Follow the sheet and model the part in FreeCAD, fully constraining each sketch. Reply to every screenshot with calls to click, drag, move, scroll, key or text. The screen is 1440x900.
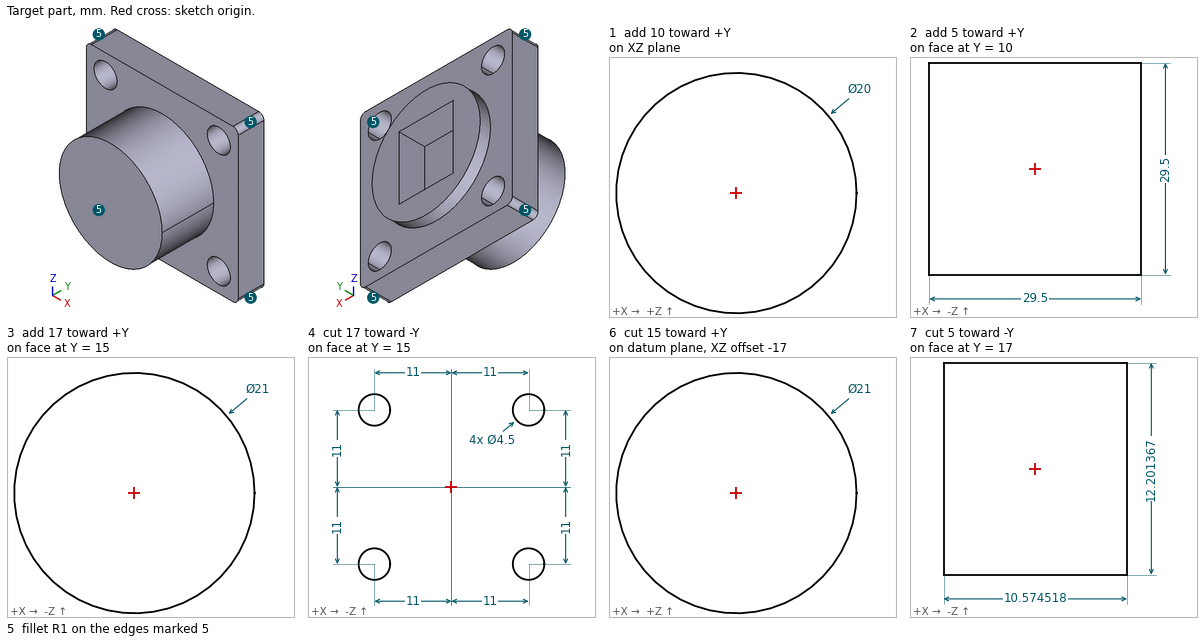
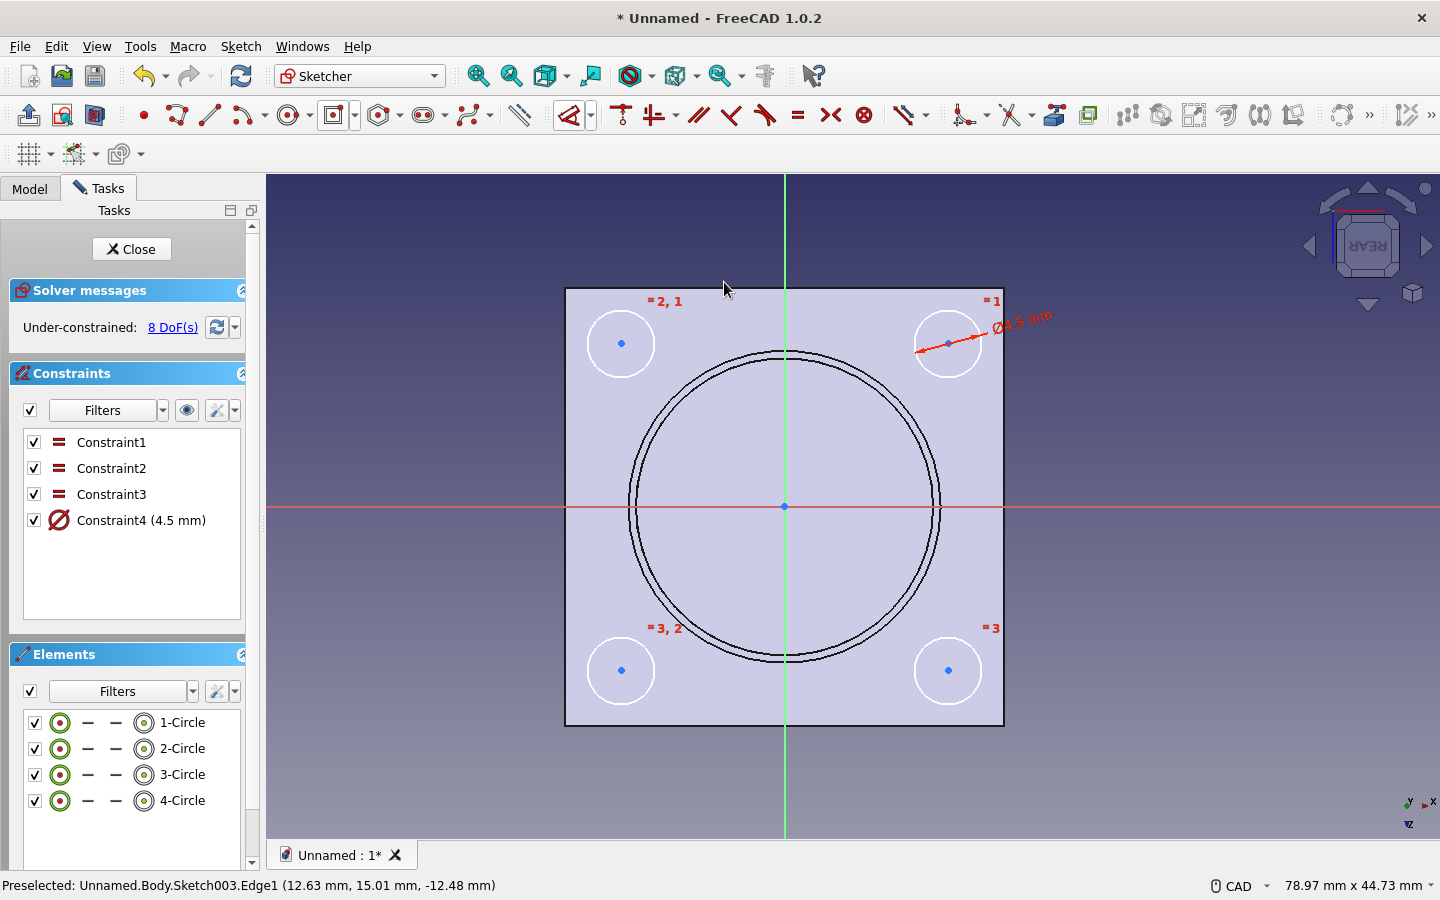
click(948, 344)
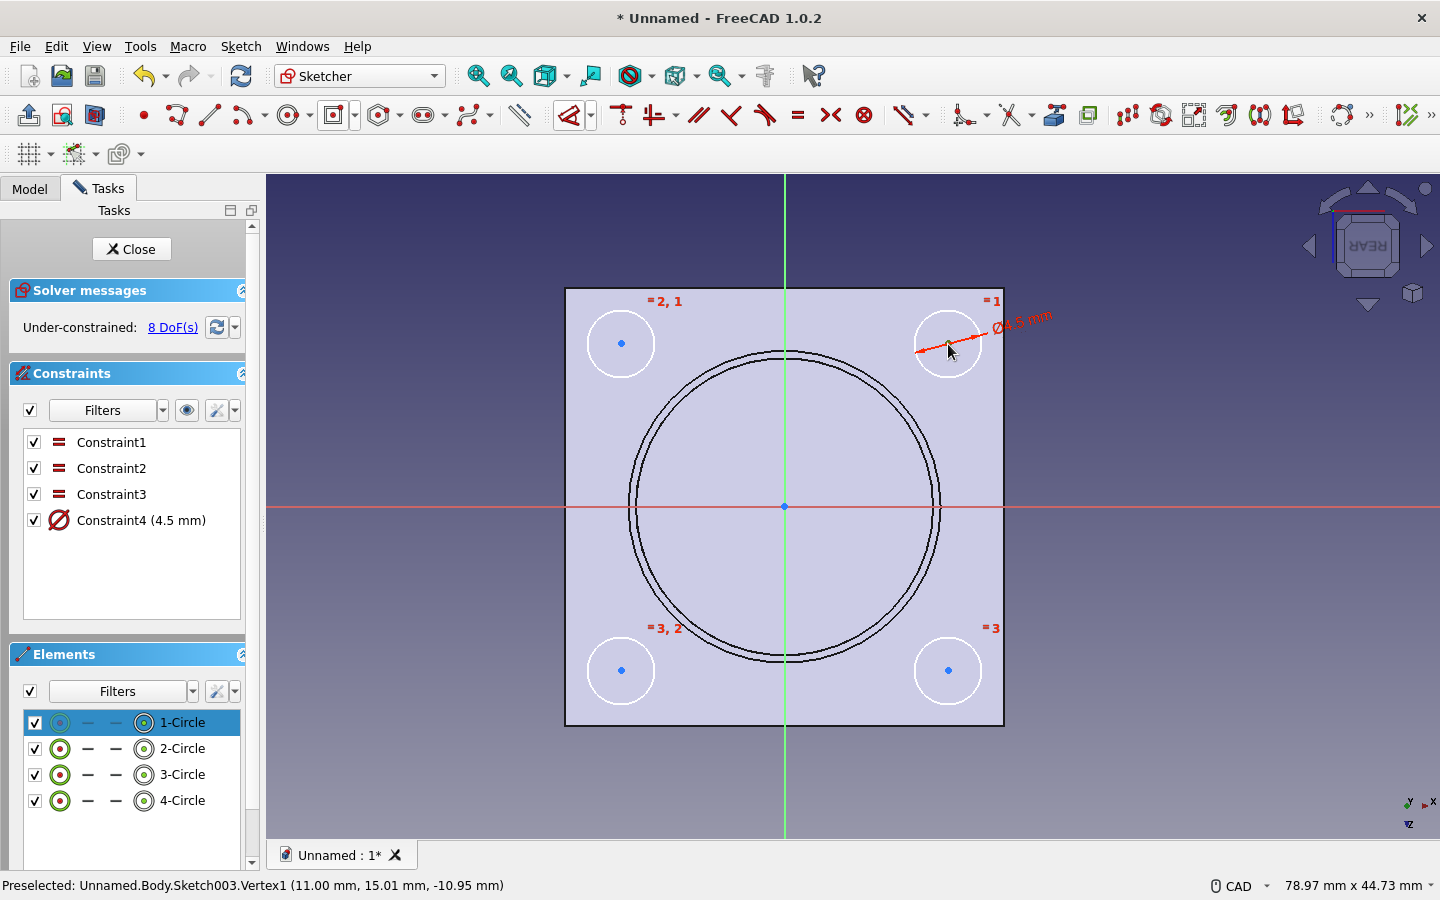
click(590, 116)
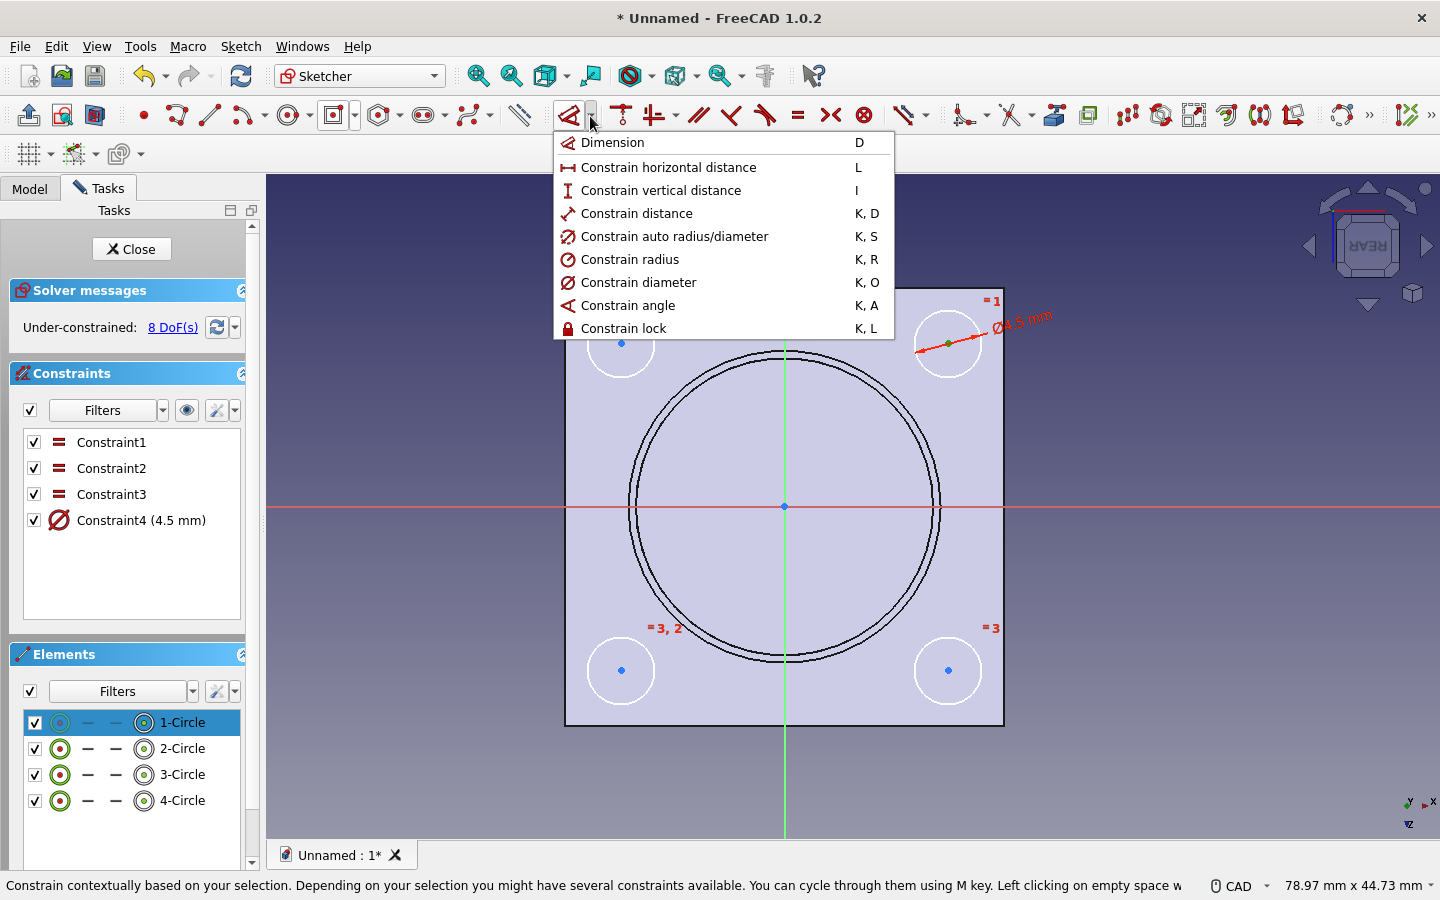
click(724, 168)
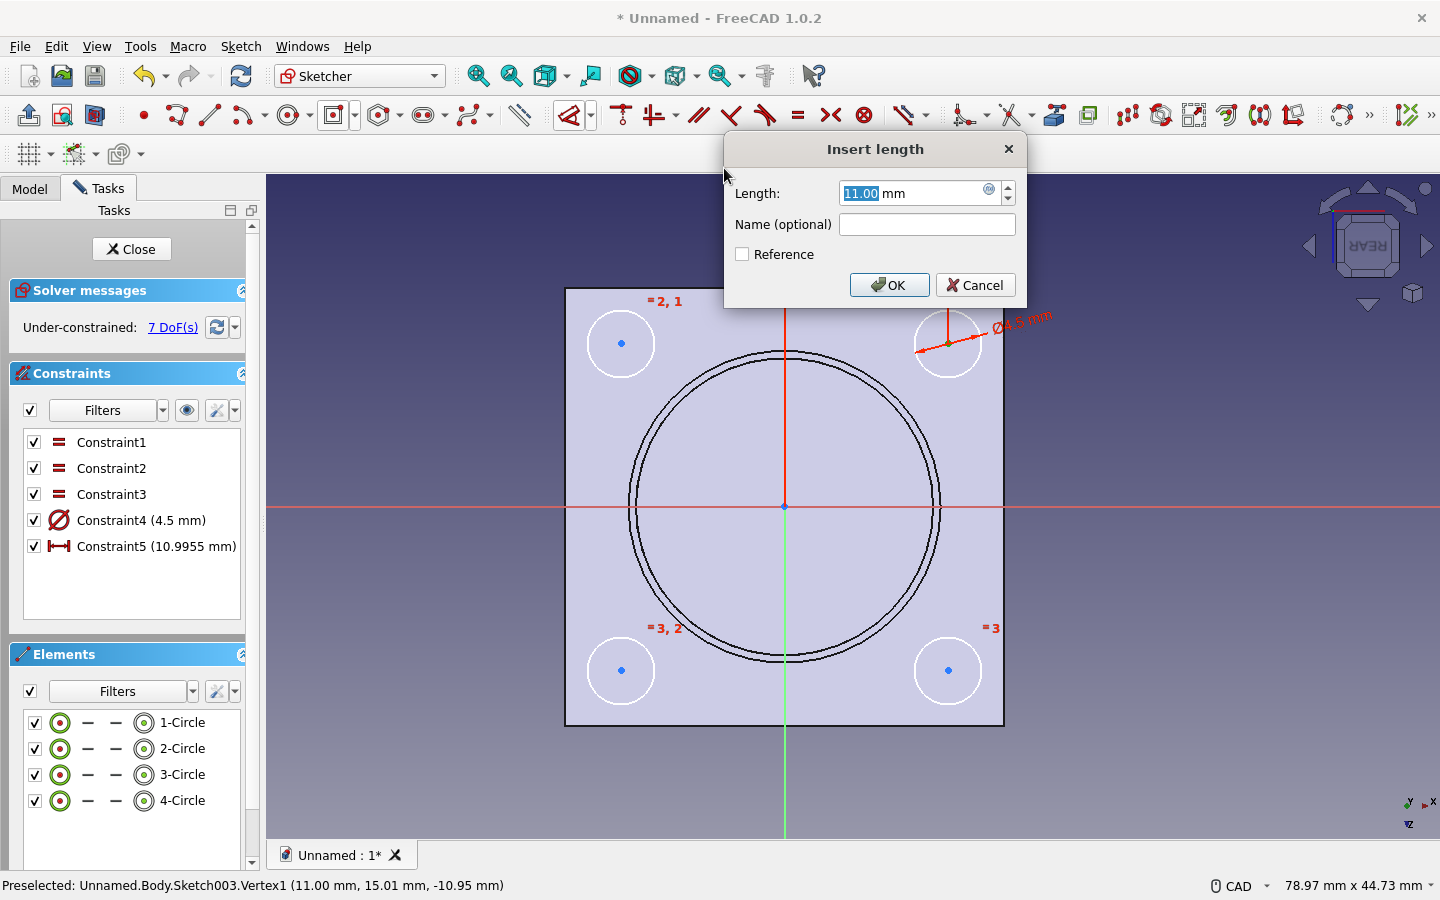
text(11)
key(Return)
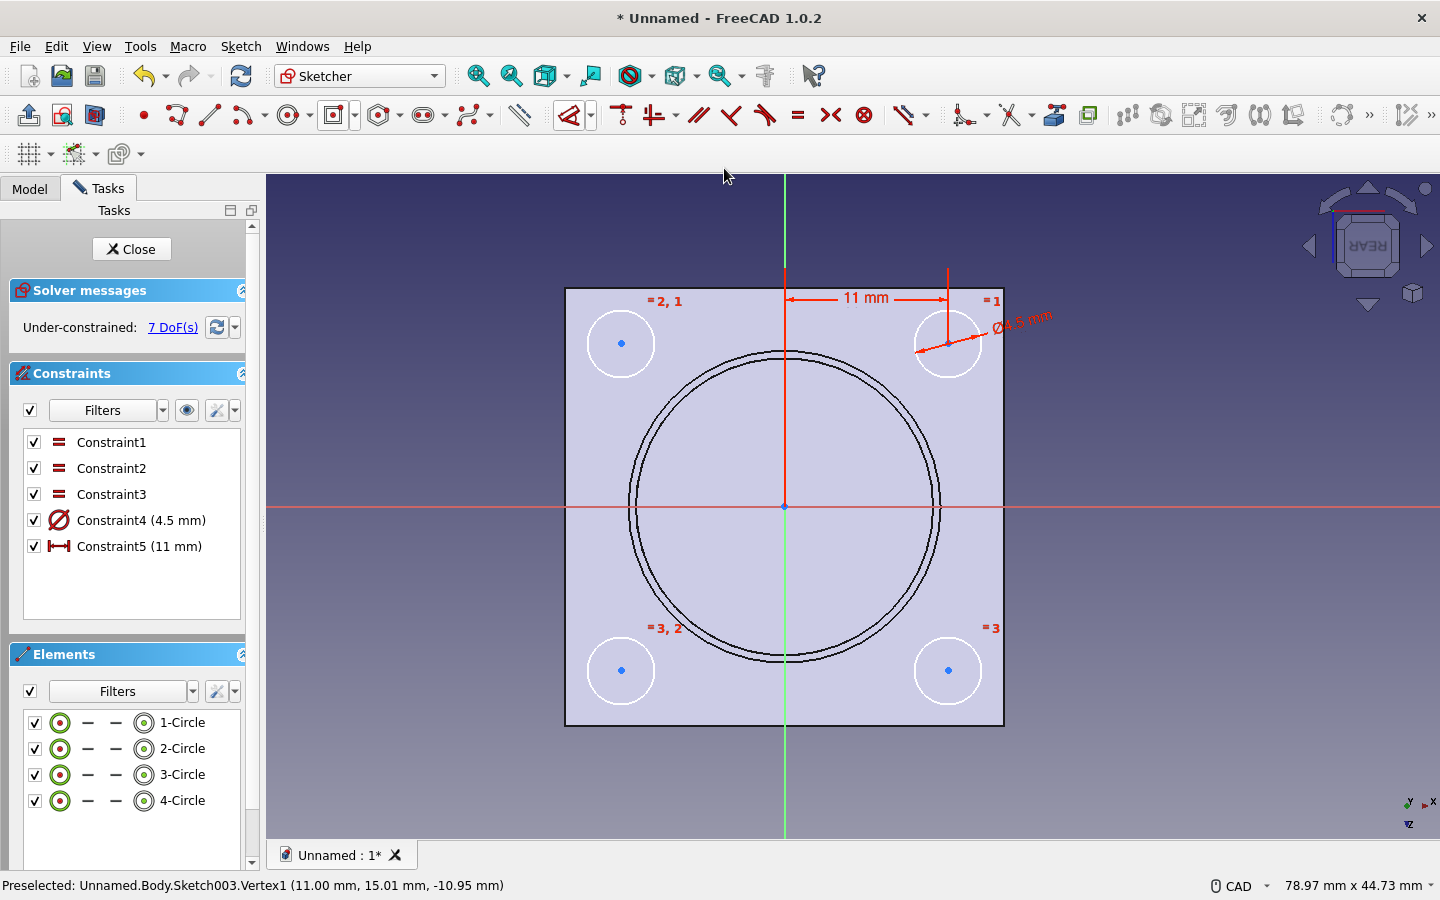
click(948, 344)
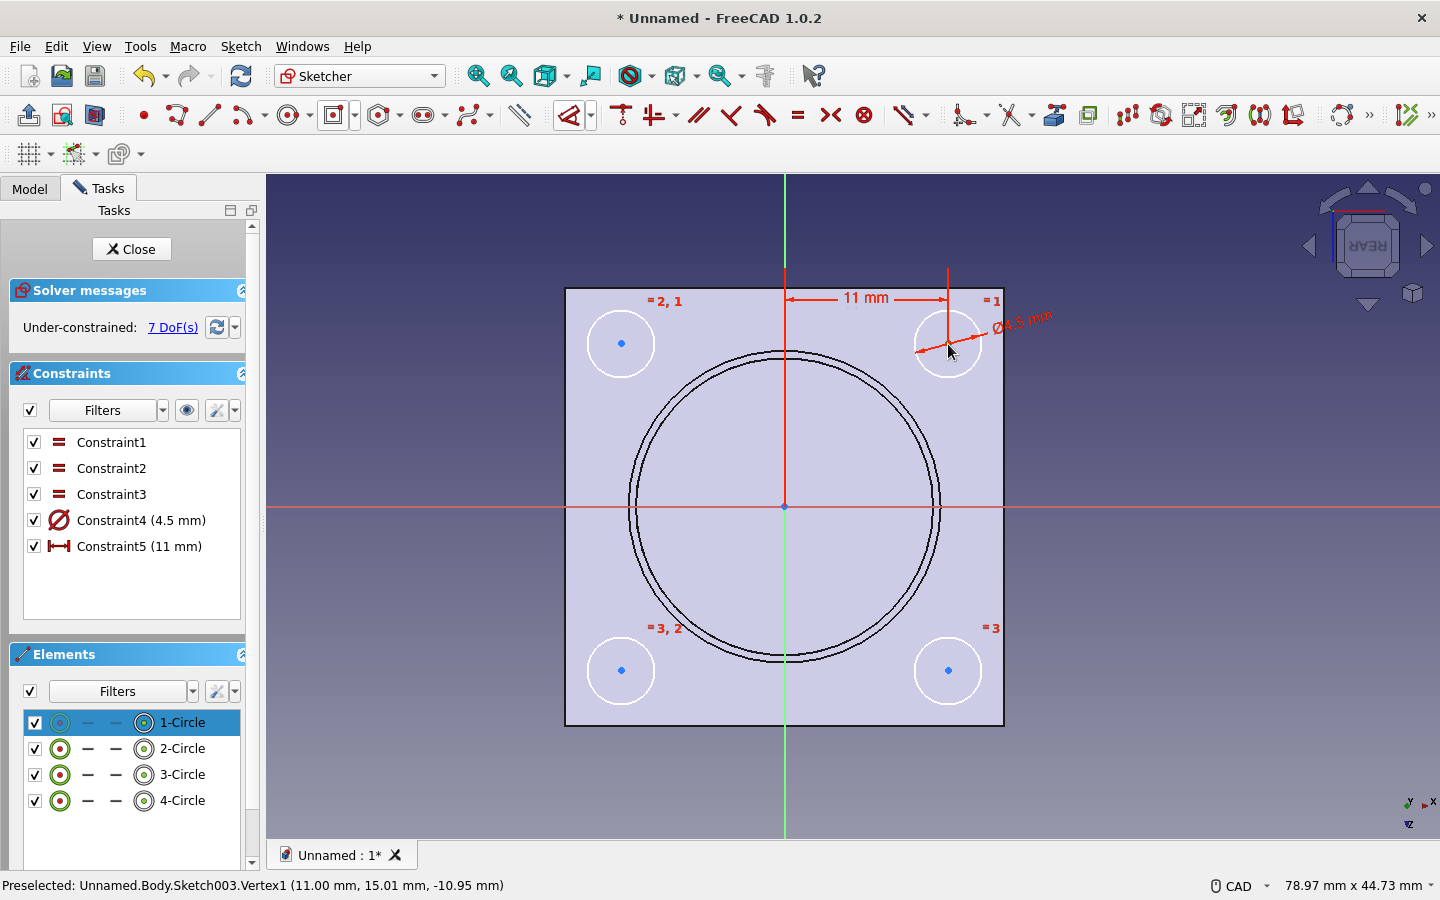
key(i)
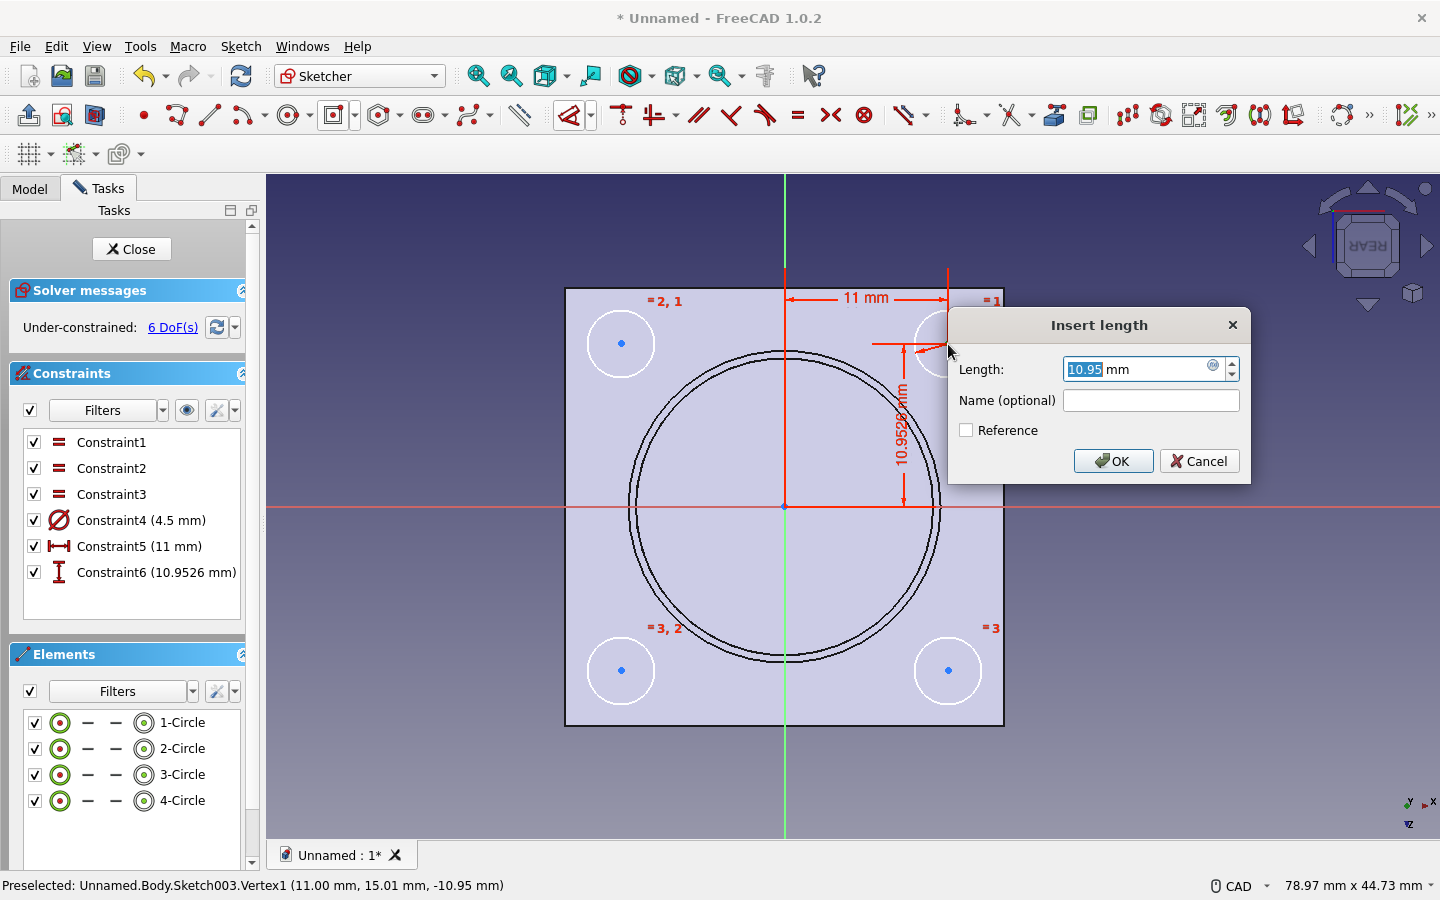
text(11)
key(Return)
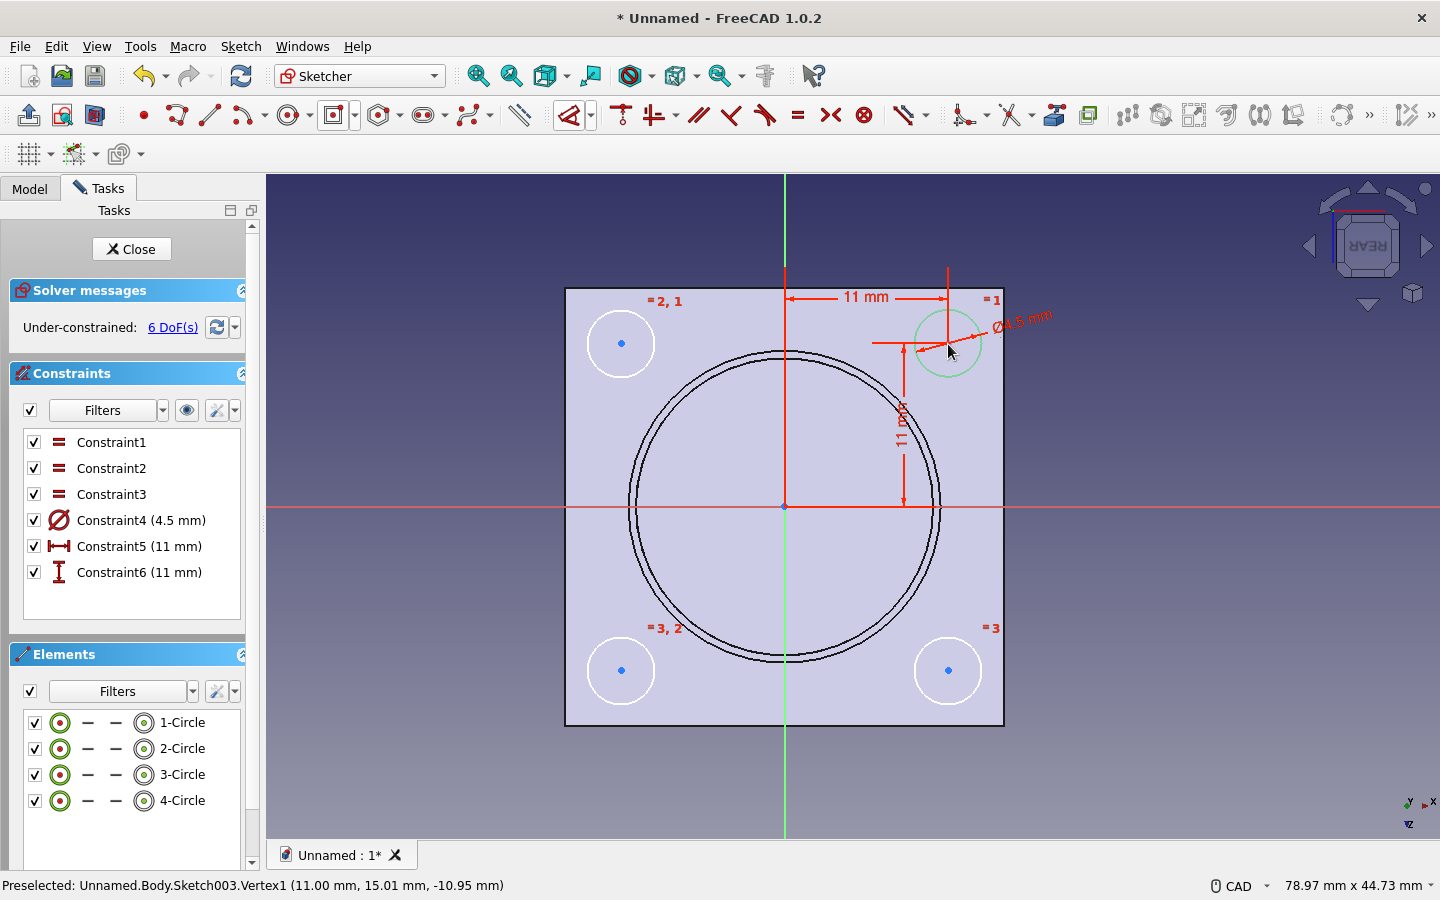
click(621, 344)